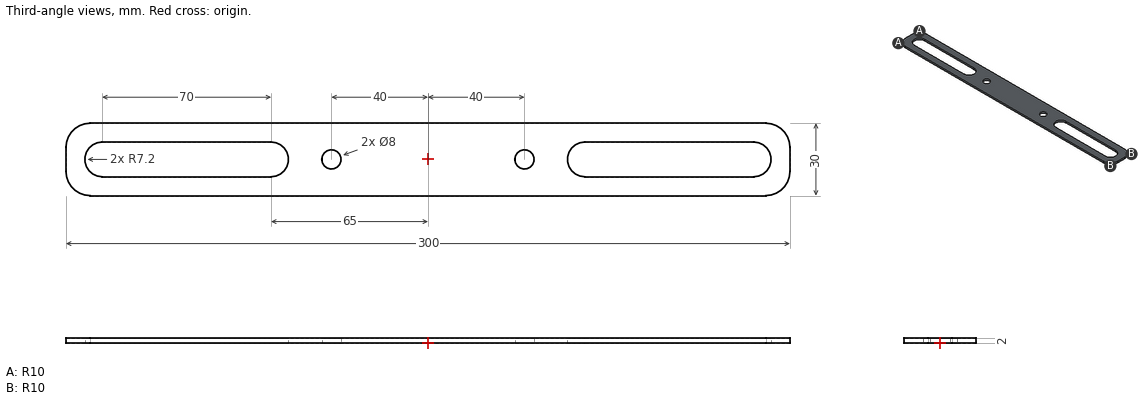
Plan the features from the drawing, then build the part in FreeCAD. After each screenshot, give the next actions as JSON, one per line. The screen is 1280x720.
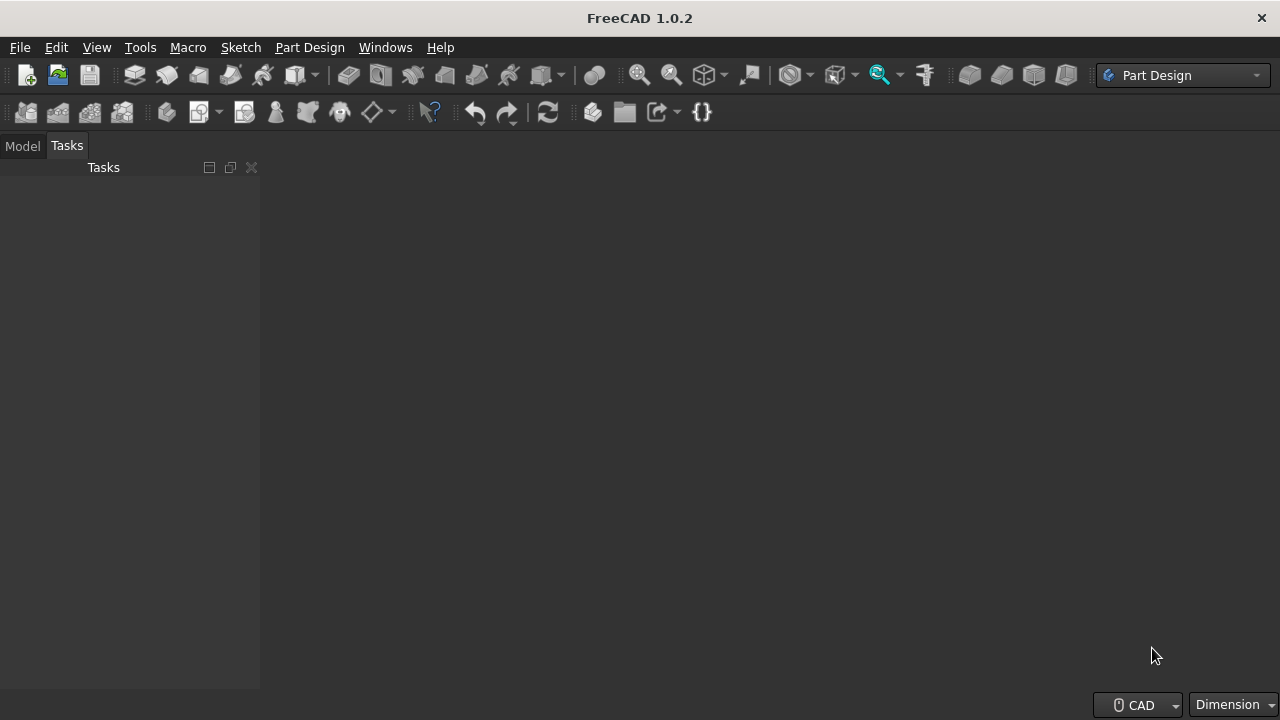
{"action": "key", "text": "ctrl+n"}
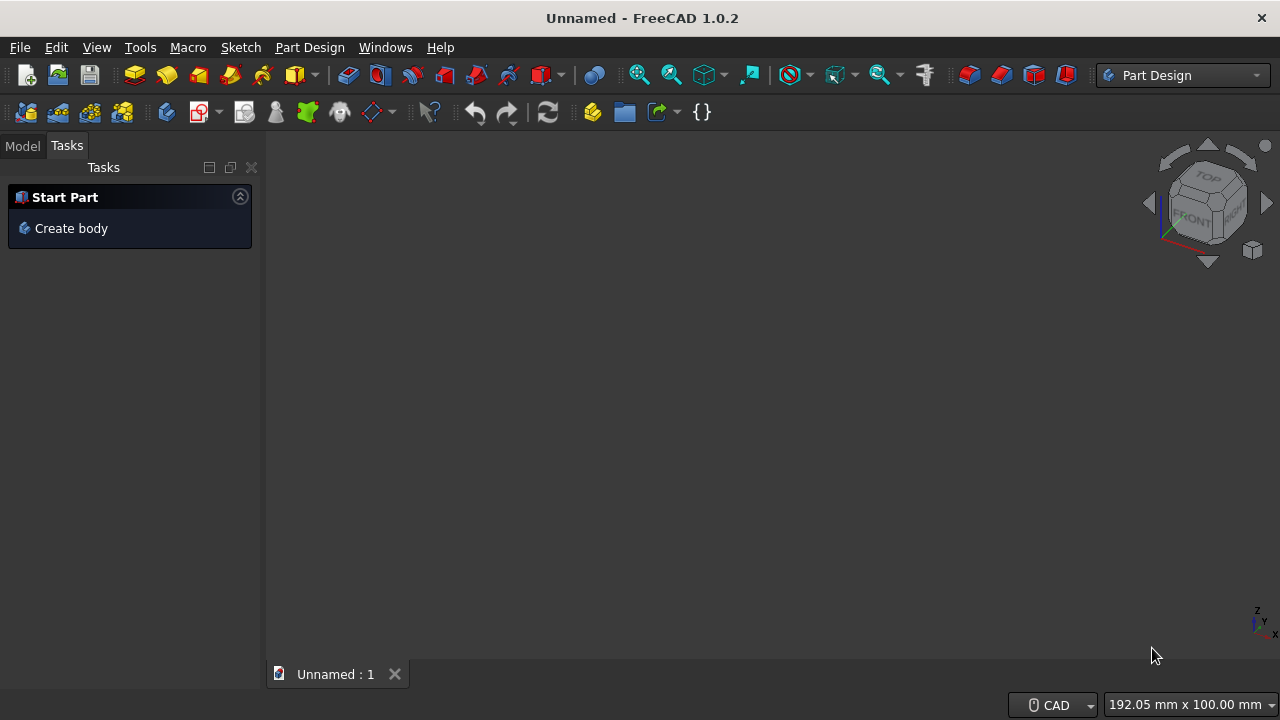
{"action": "left_click", "coordinate": [200, 112]}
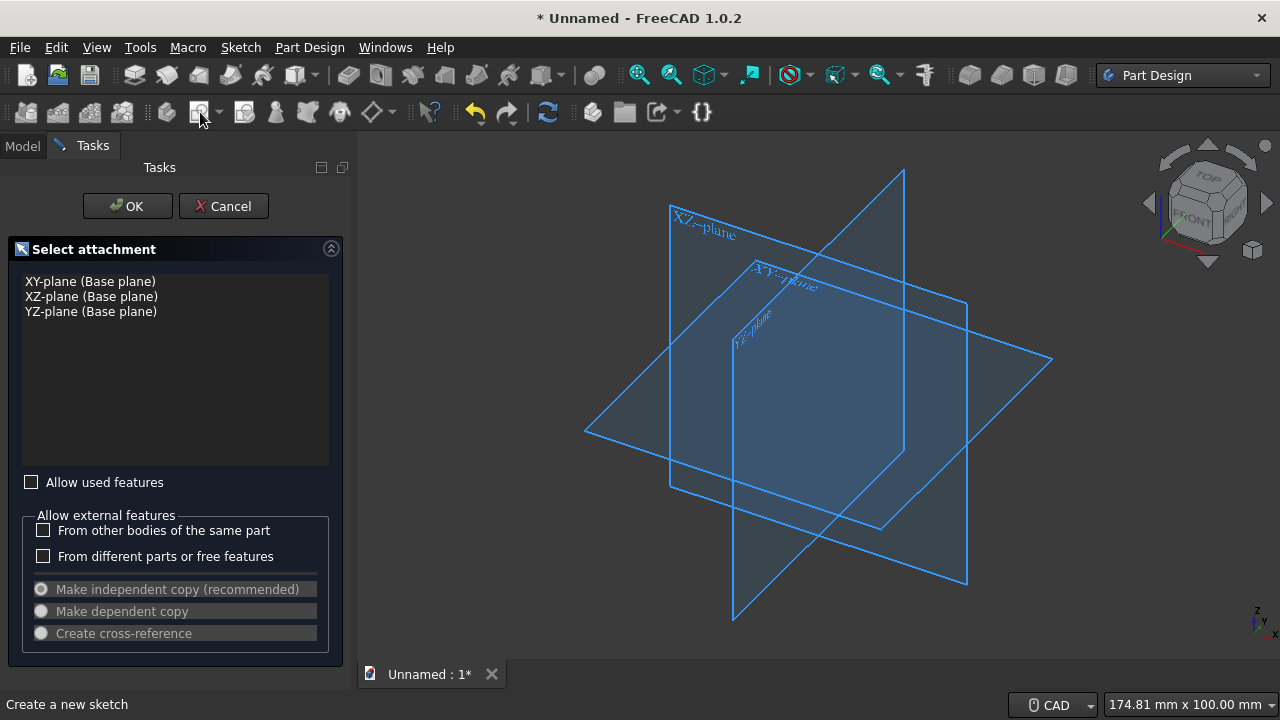
{"action": "left_click", "coordinate": [82, 282]}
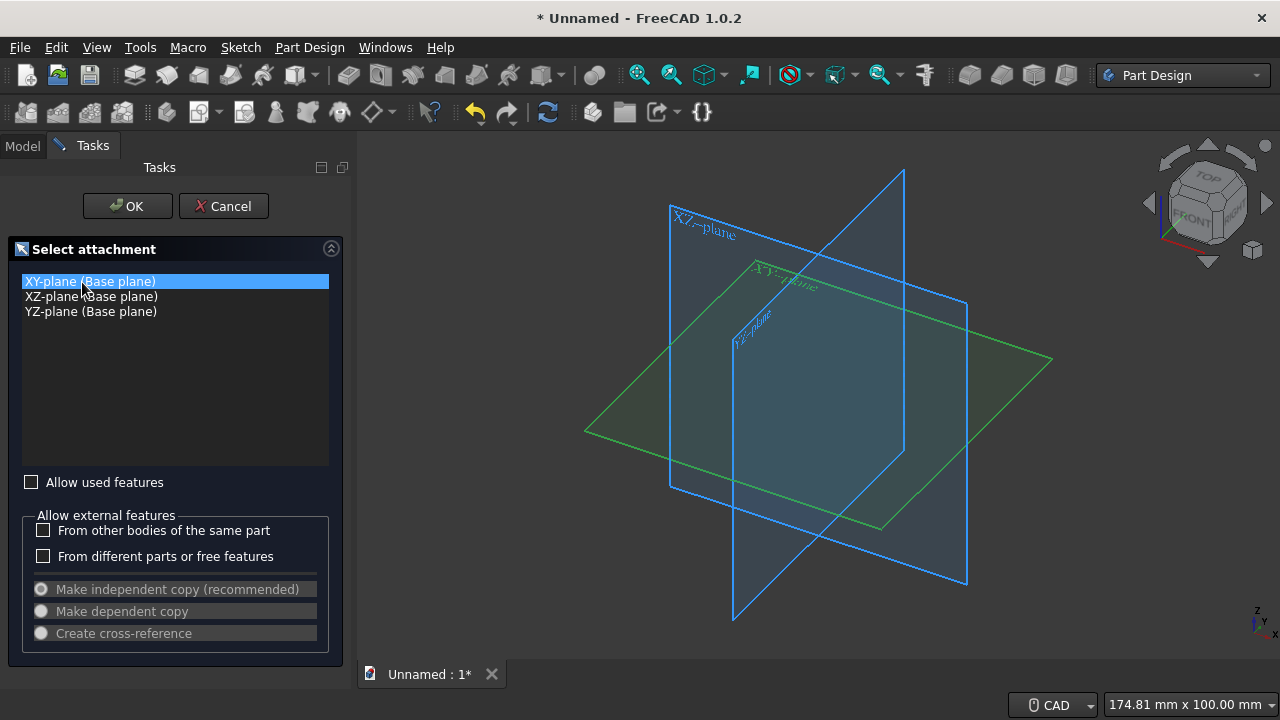
{"action": "left_click", "coordinate": [128, 206]}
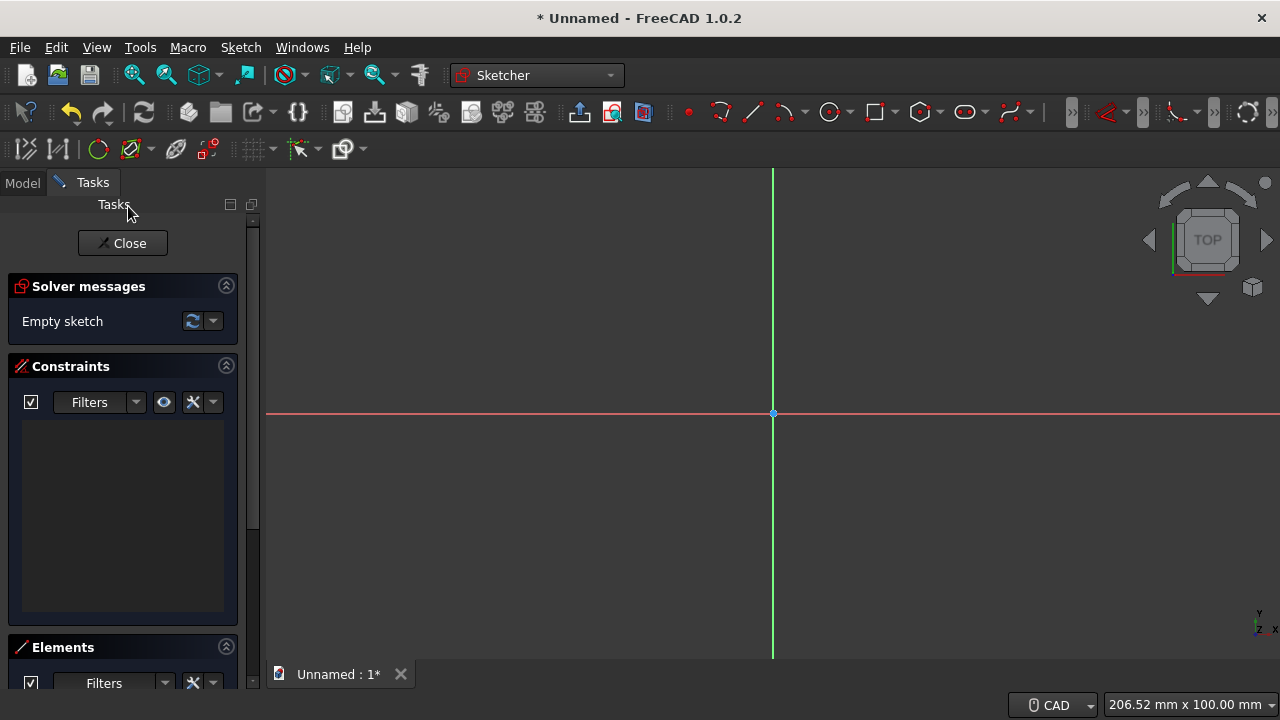
{"action": "scroll", "coordinate": [665, 414], "scroll_direction": "down", "scroll_amount": 5}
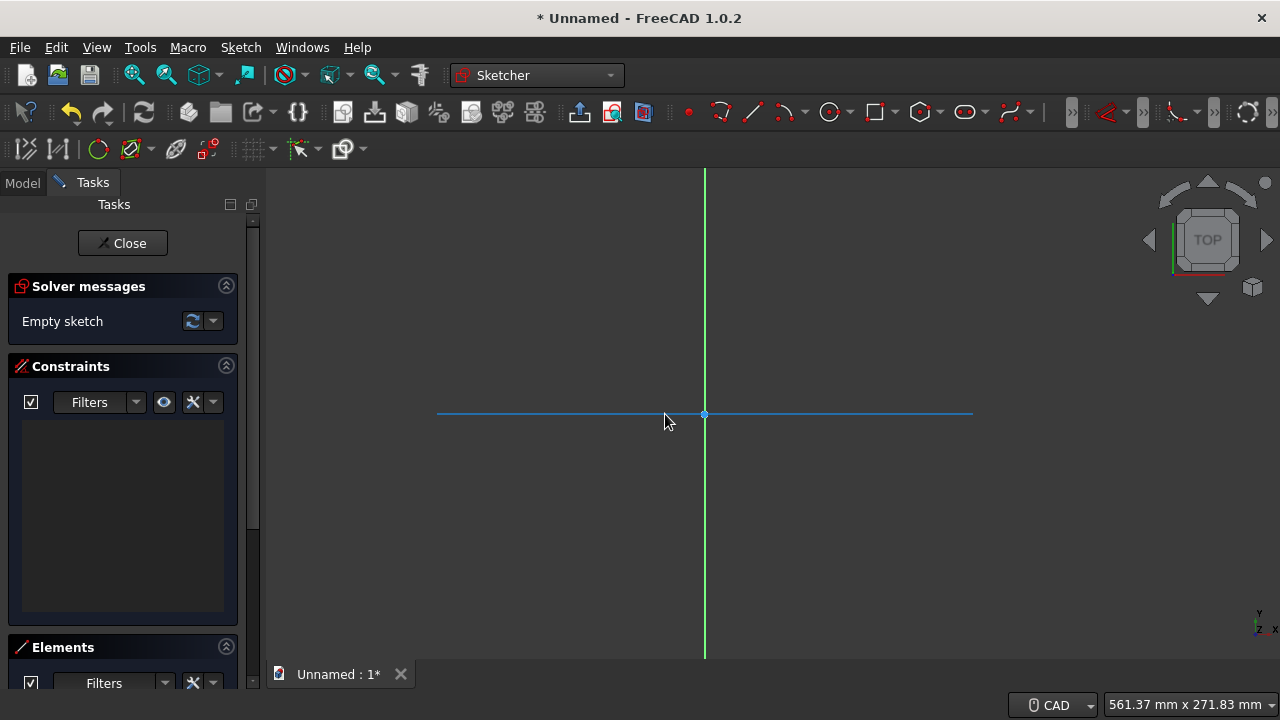
{"action": "key", "text": "g v"}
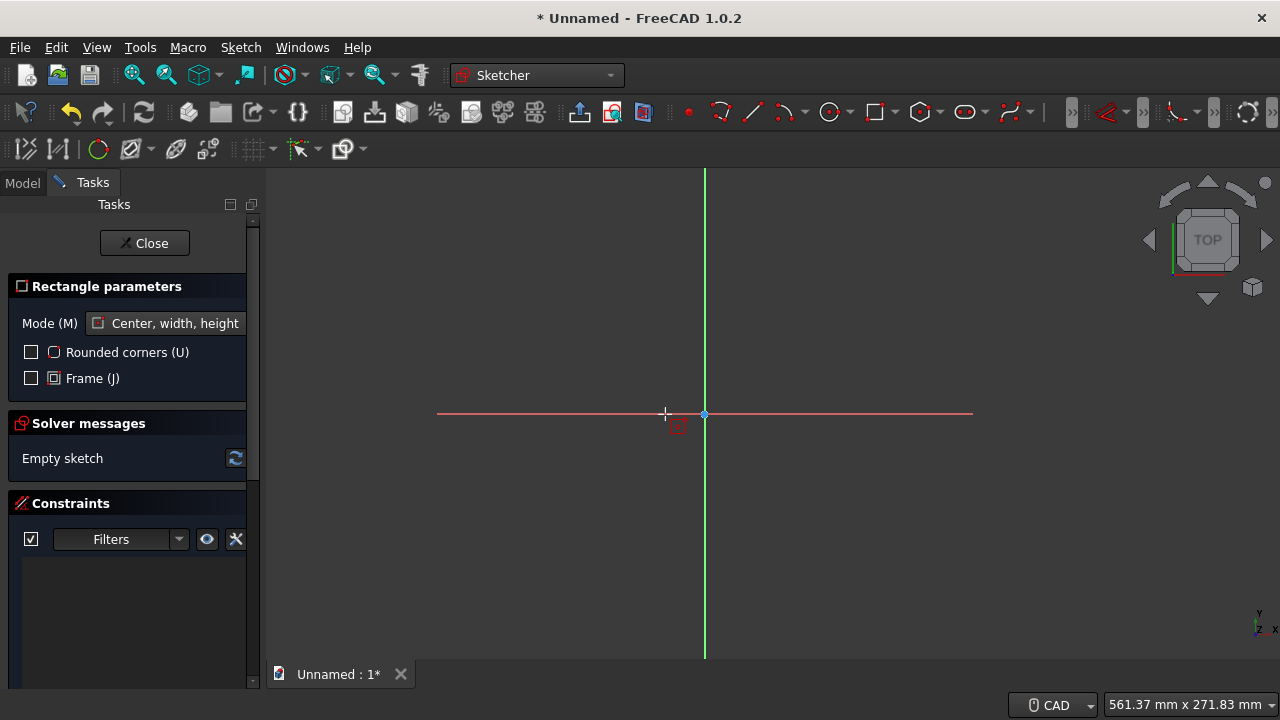
{"action": "left_click", "coordinate": [705, 414]}
{"action": "left_click", "coordinate": [976, 387]}
{"action": "key", "text": "Escape"}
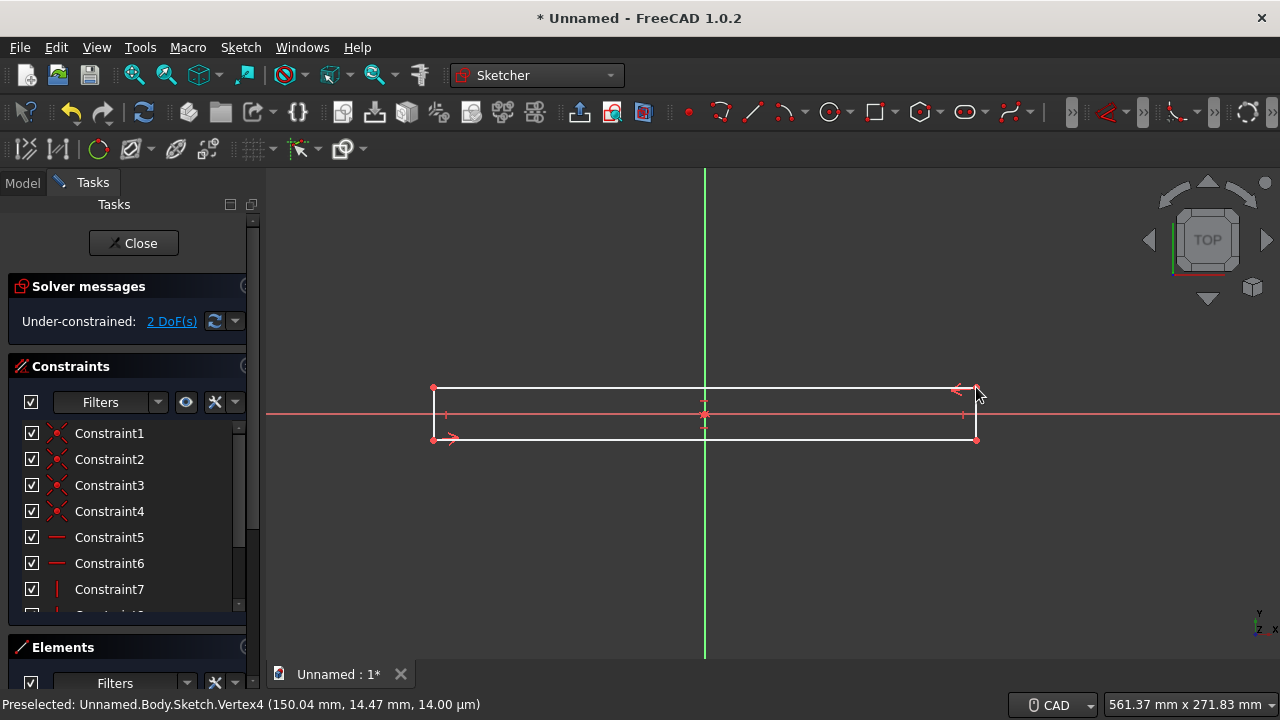
{"action": "scroll", "coordinate": [976, 425], "scroll_direction": "up", "scroll_amount": 2}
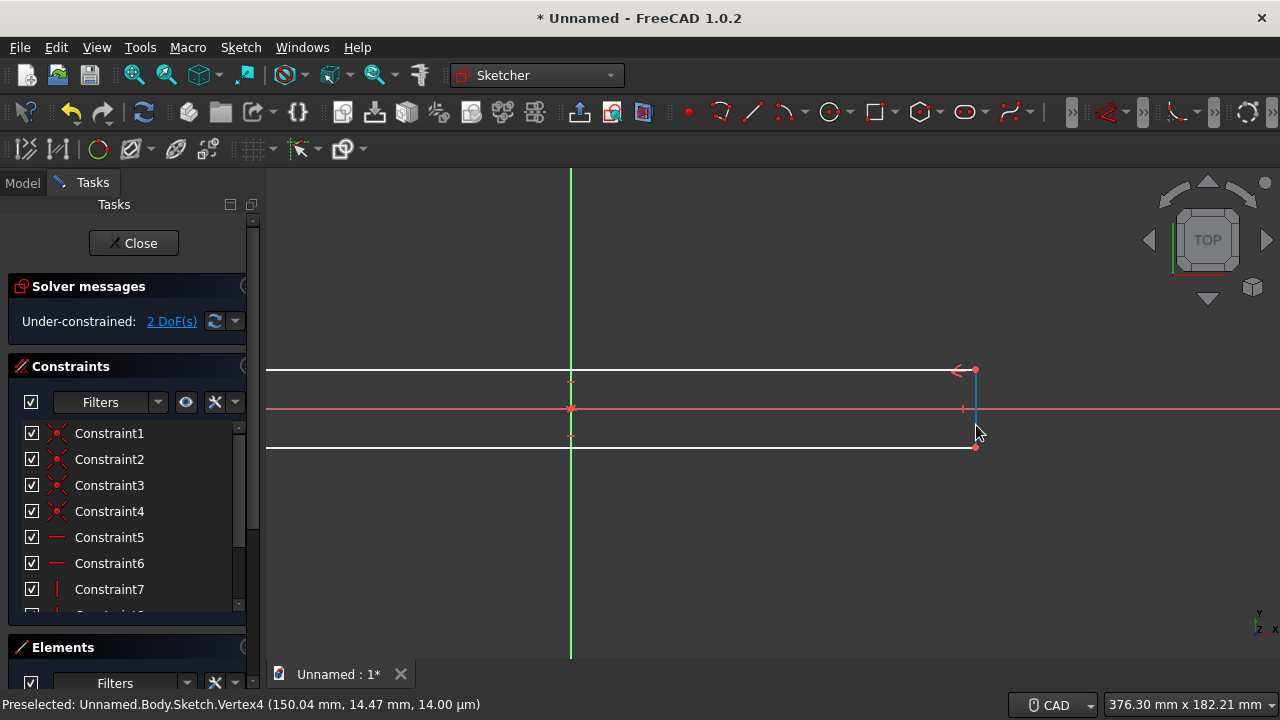
{"action": "left_click", "coordinate": [976, 424]}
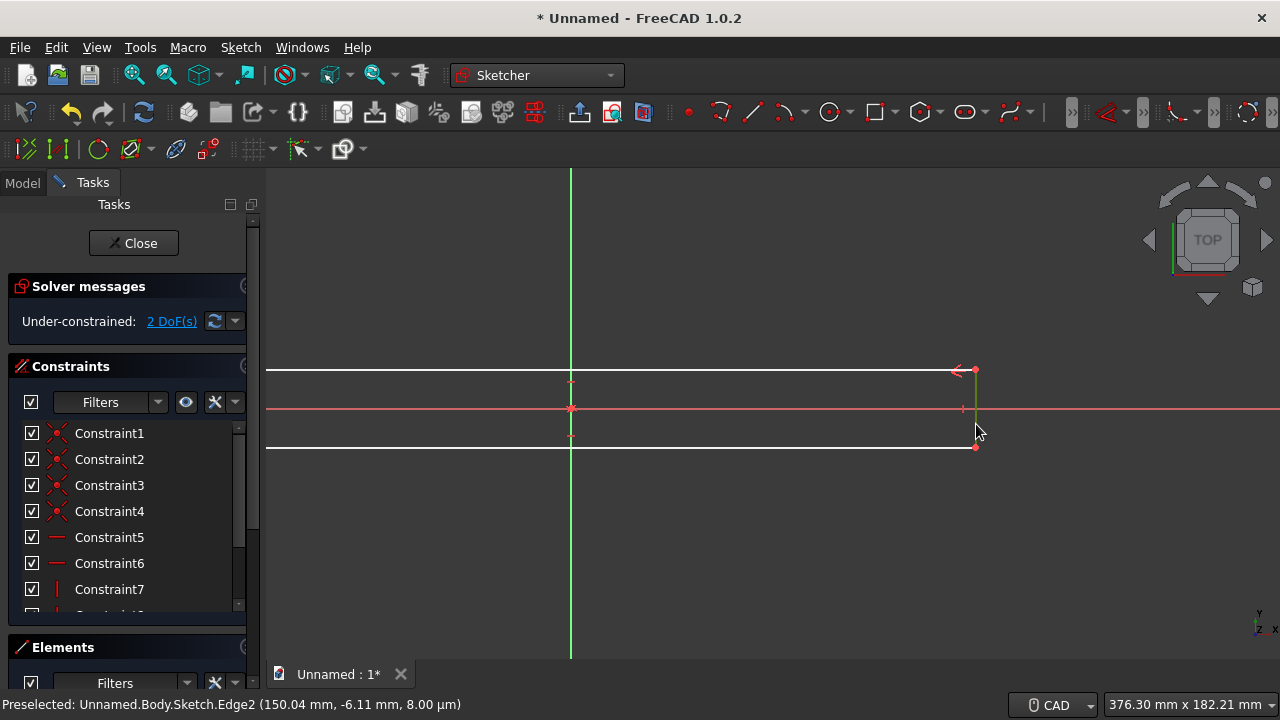
{"action": "key", "text": "i"}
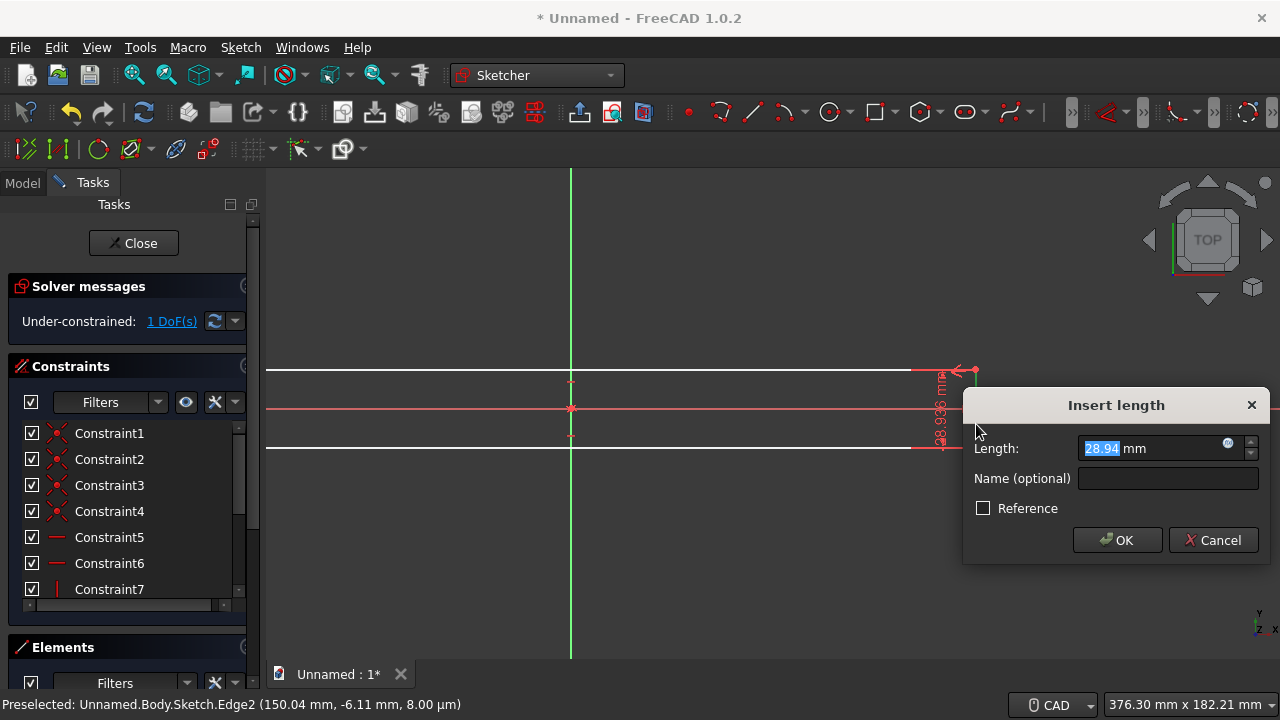
{"action": "type", "text": "30"}
{"action": "key", "text": "Return"}